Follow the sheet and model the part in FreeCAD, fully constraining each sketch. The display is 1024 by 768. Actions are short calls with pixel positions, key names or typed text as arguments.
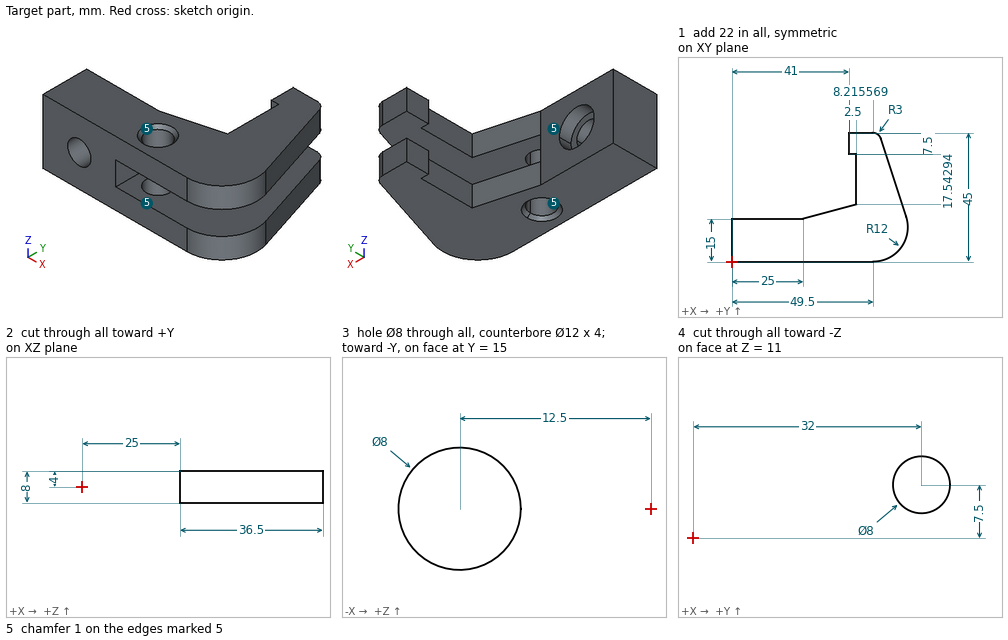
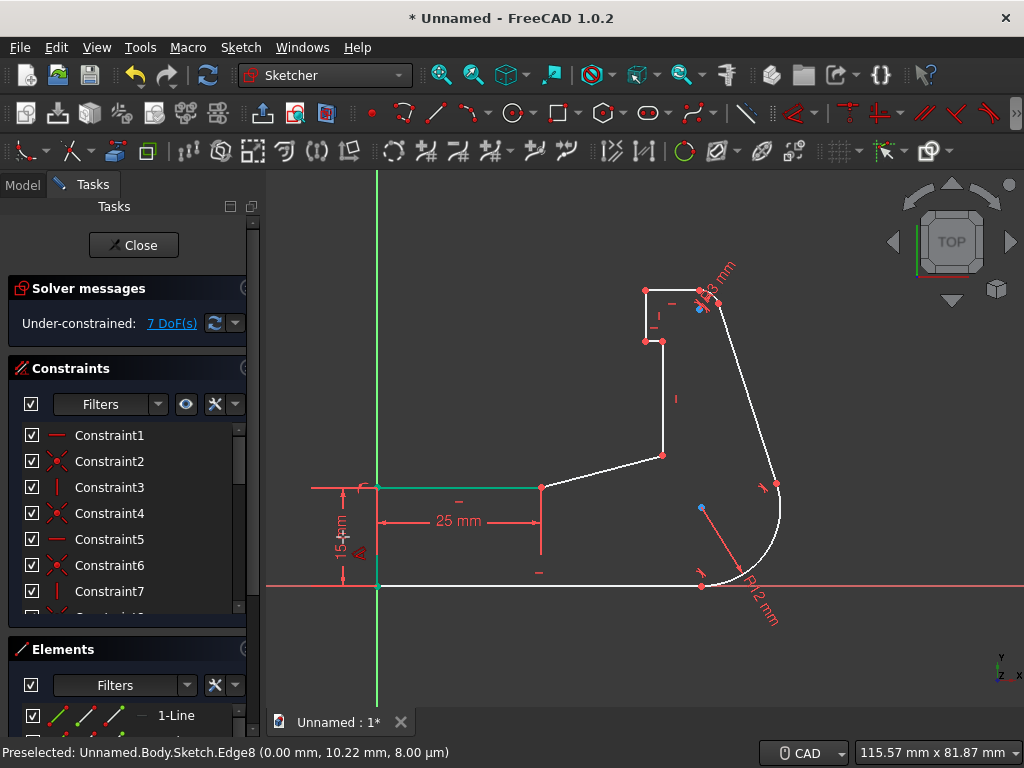
click(646, 305)
click(680, 316)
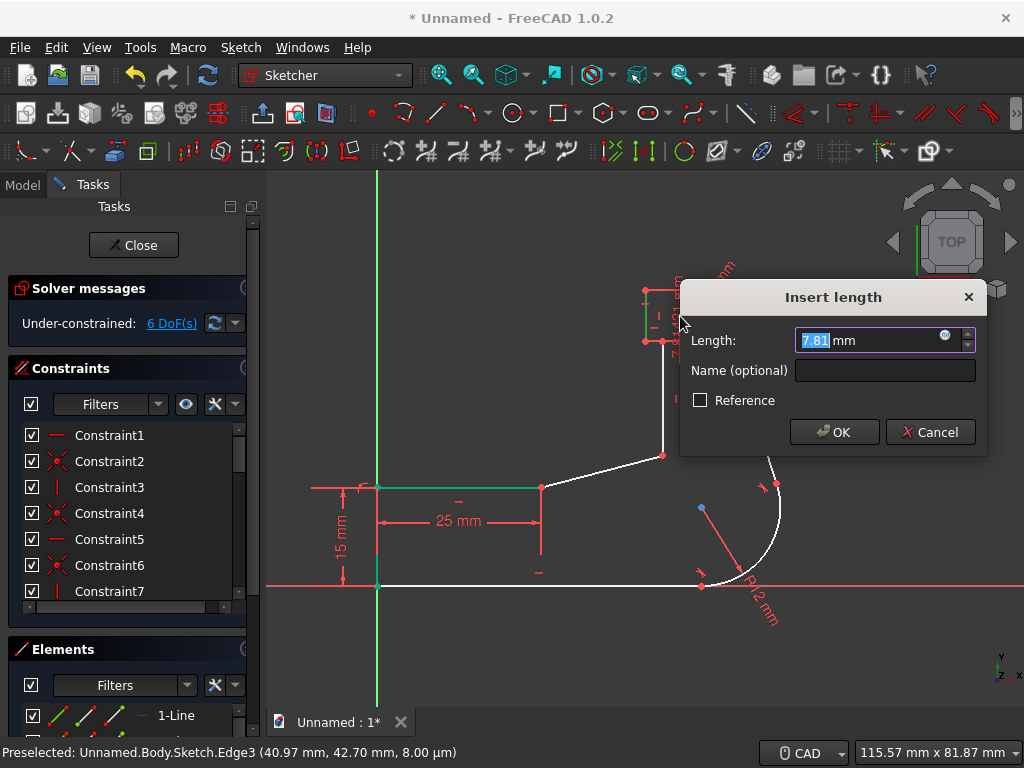
text(7.5)
key(Return)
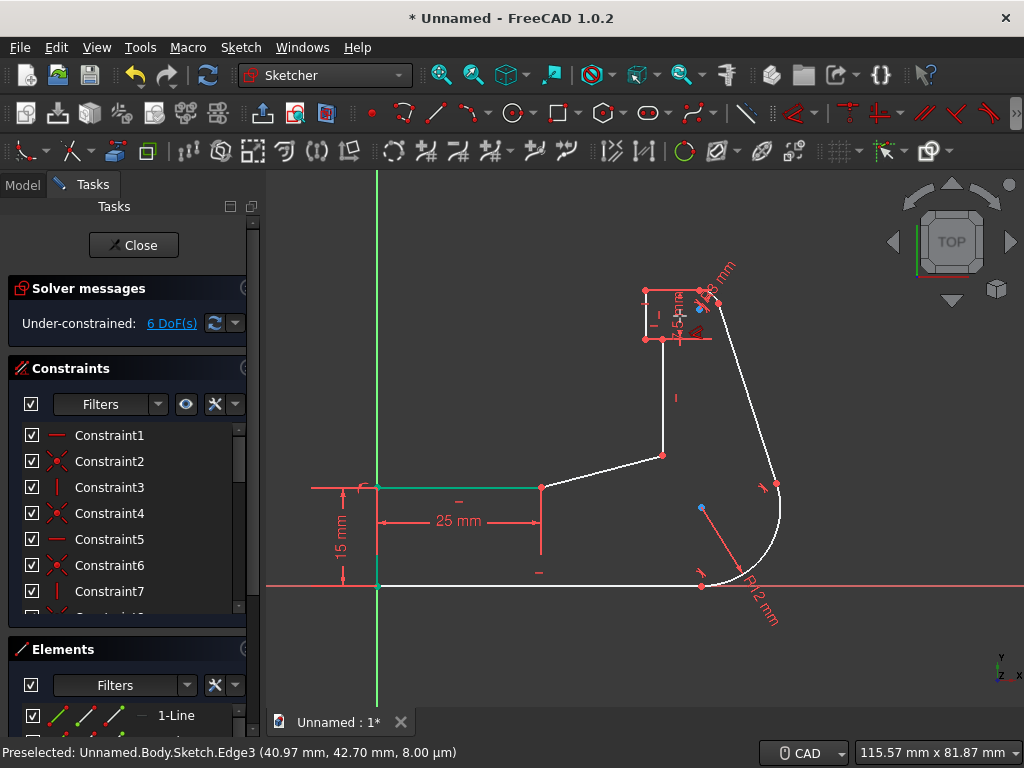
scroll(654, 339, up, 5)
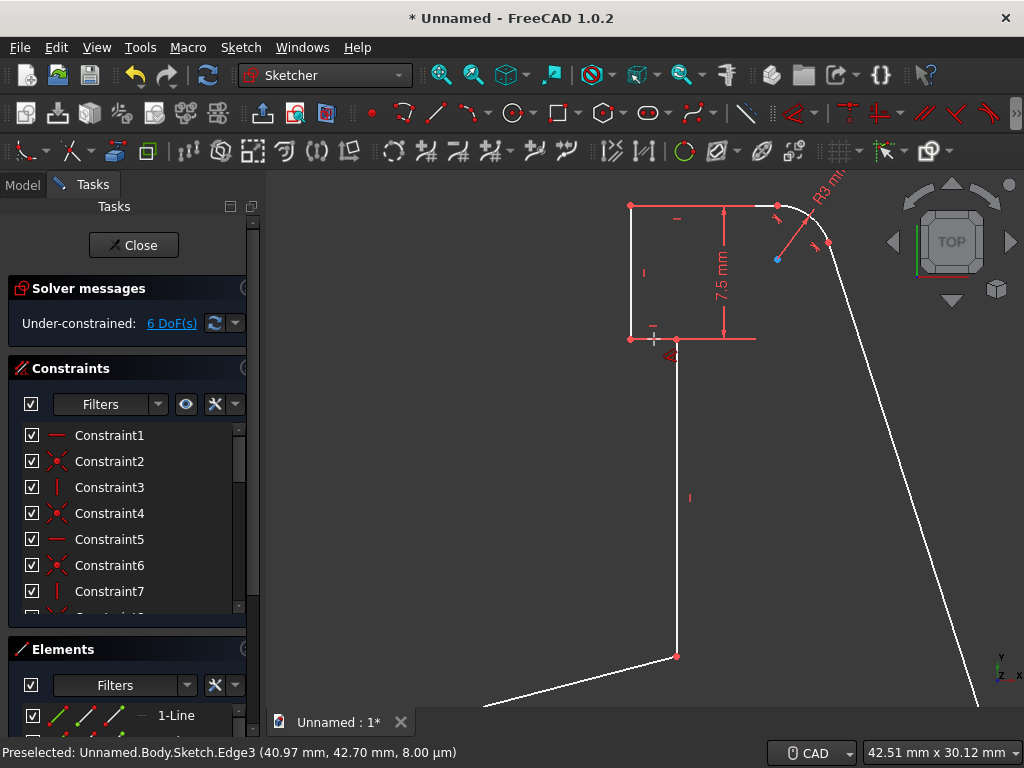
click(654, 339)
click(654, 305)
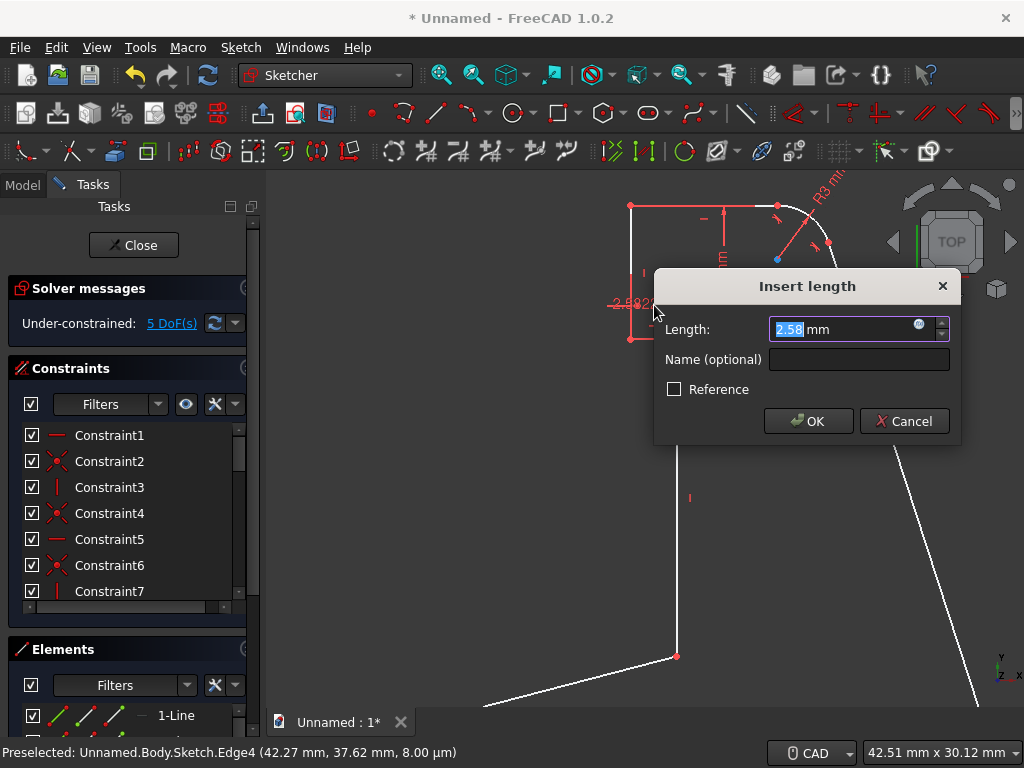
text(2.5)
key(Return)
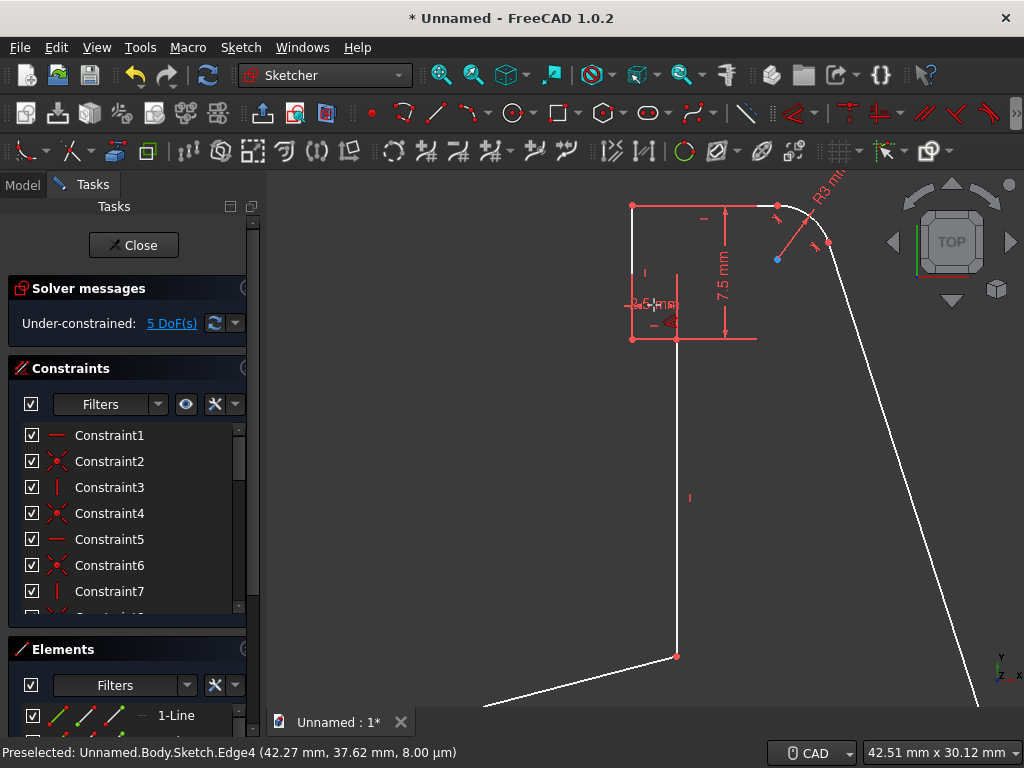
click(778, 206)
click(812, 442)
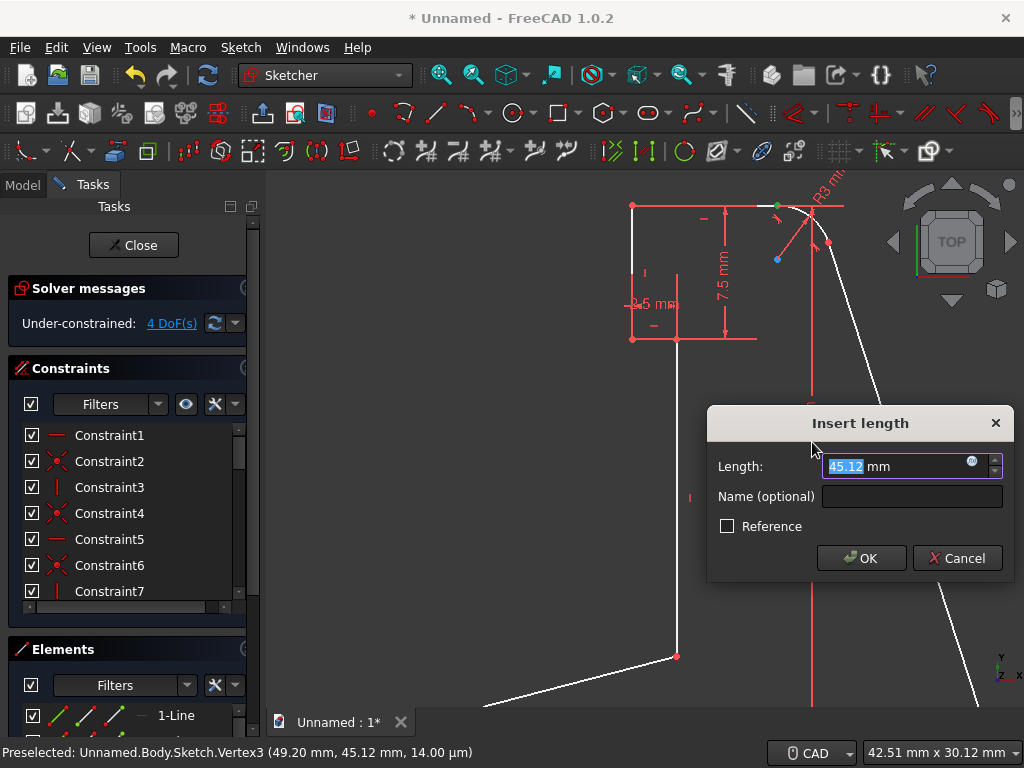
text(45)
key(Return)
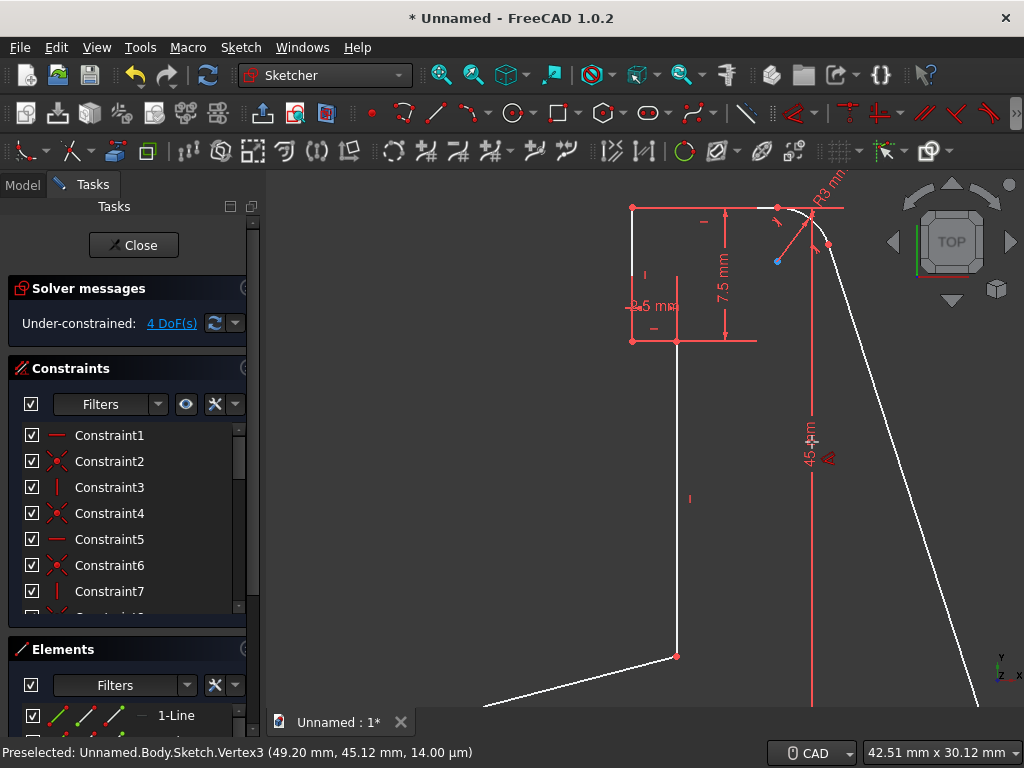
click(632, 208)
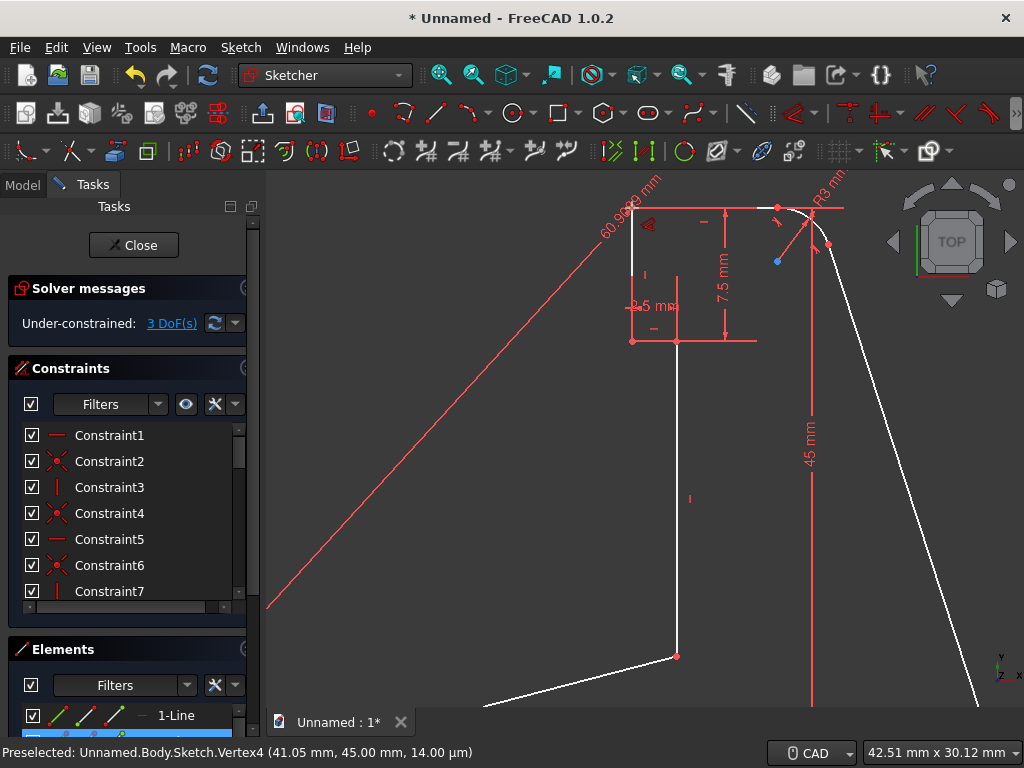
key(Escape)
key(Escape)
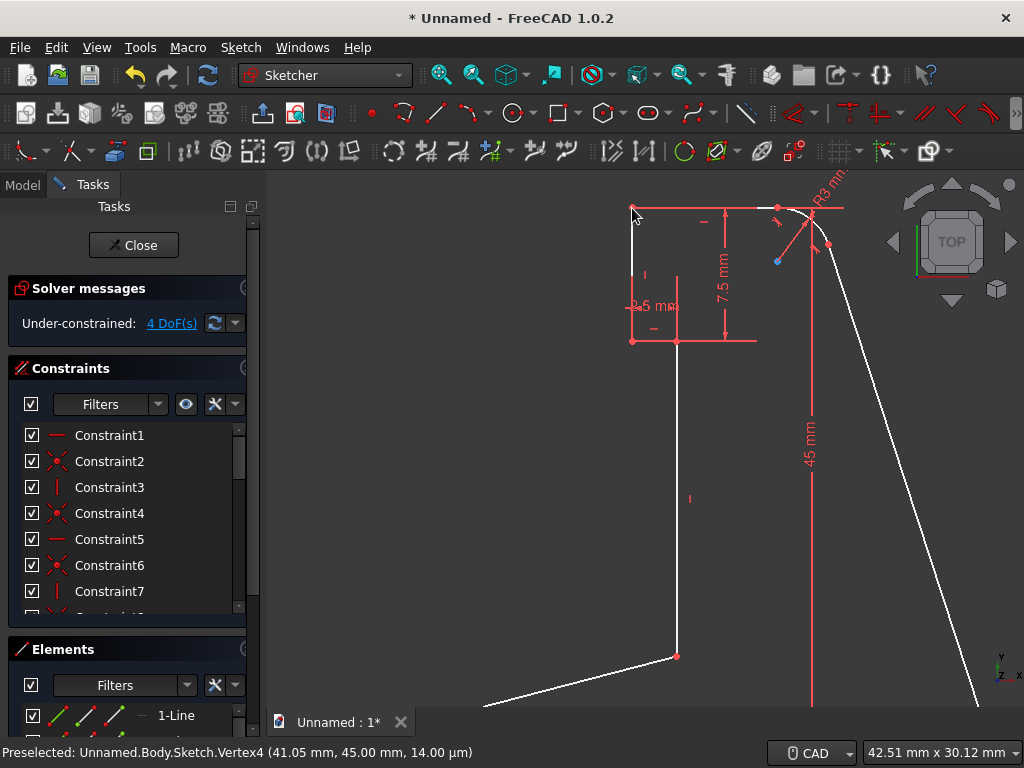
click(632, 208)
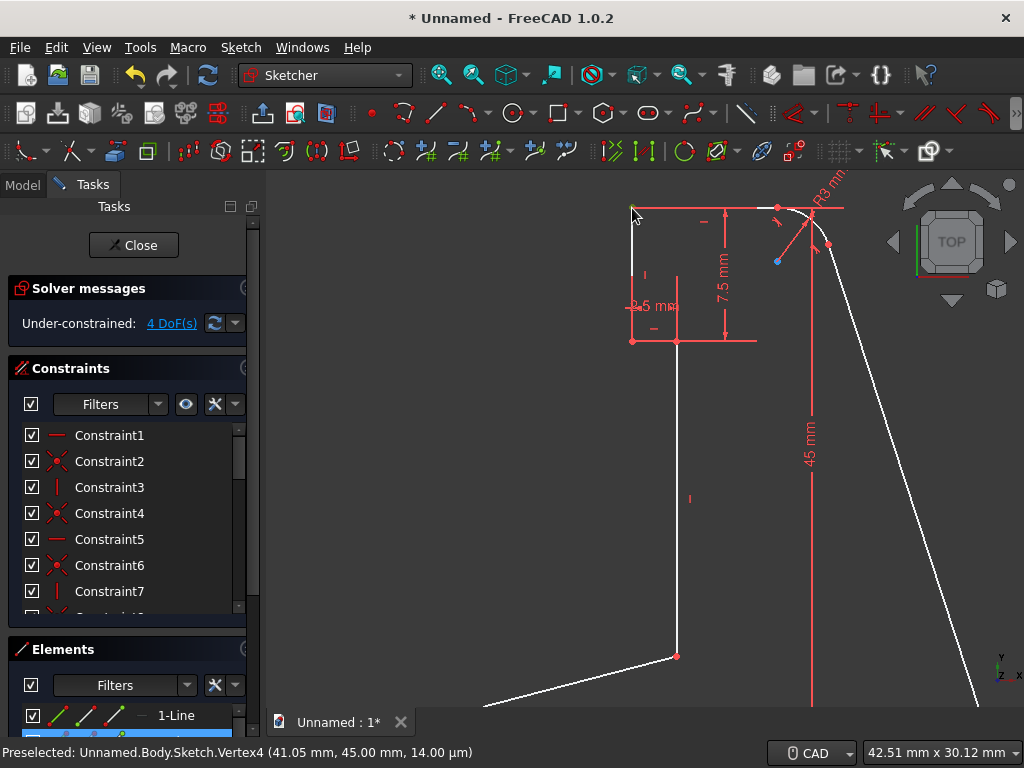
key(l)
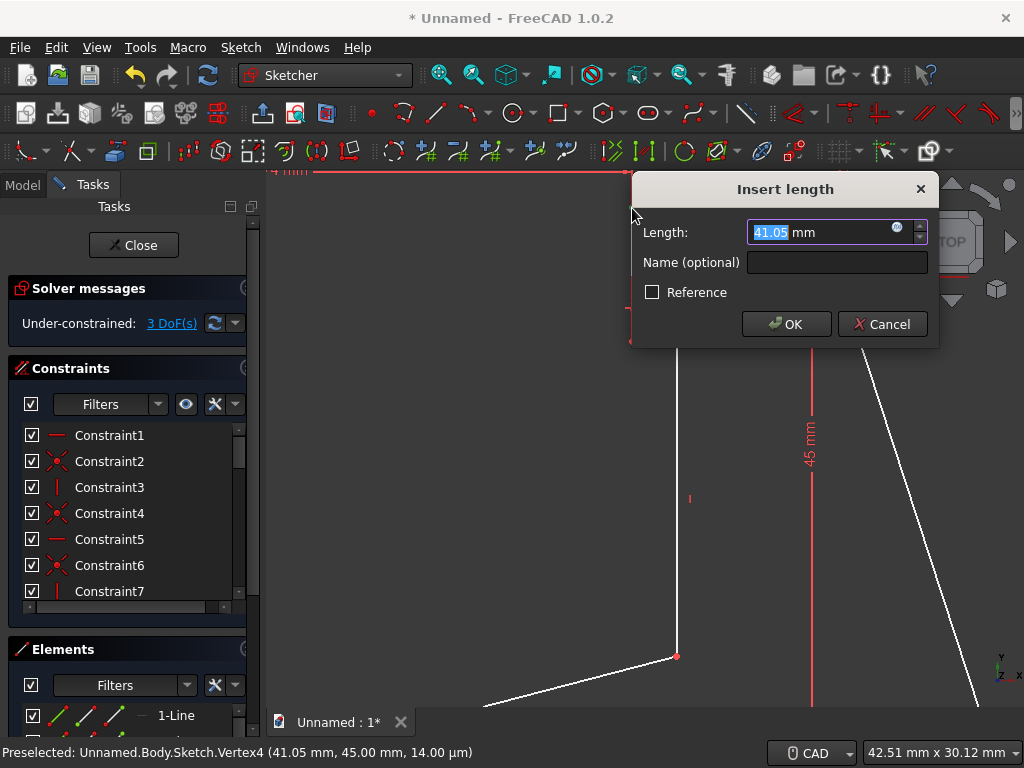
text(41)
key(Return)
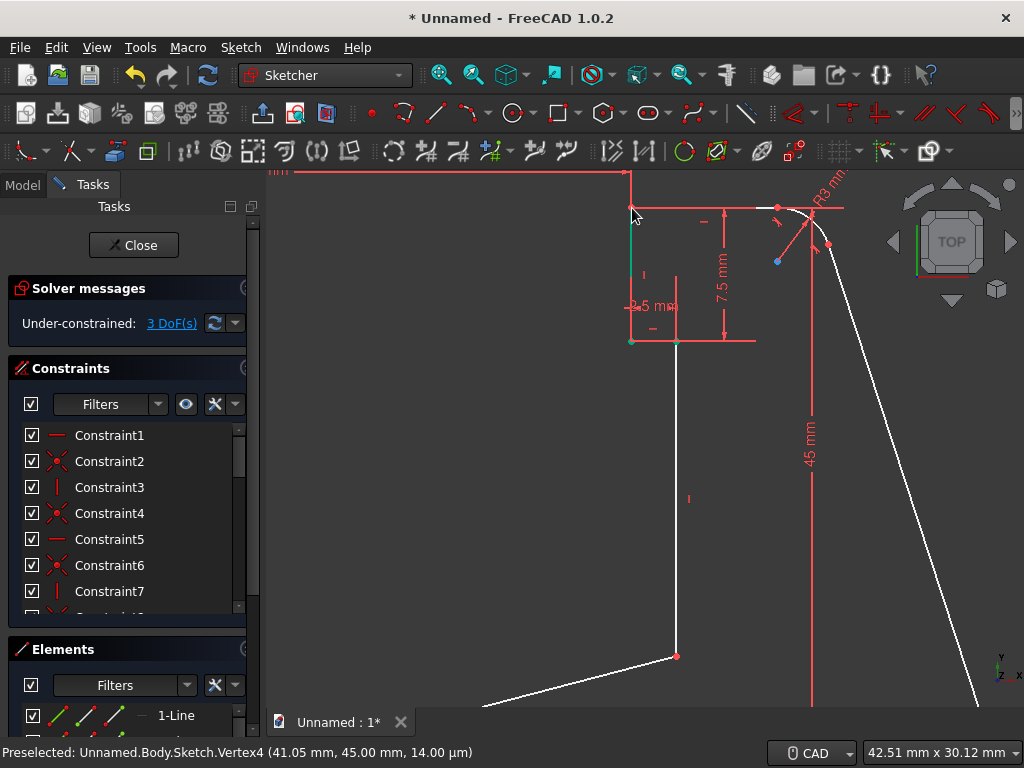
scroll(654, 339, down, 5)